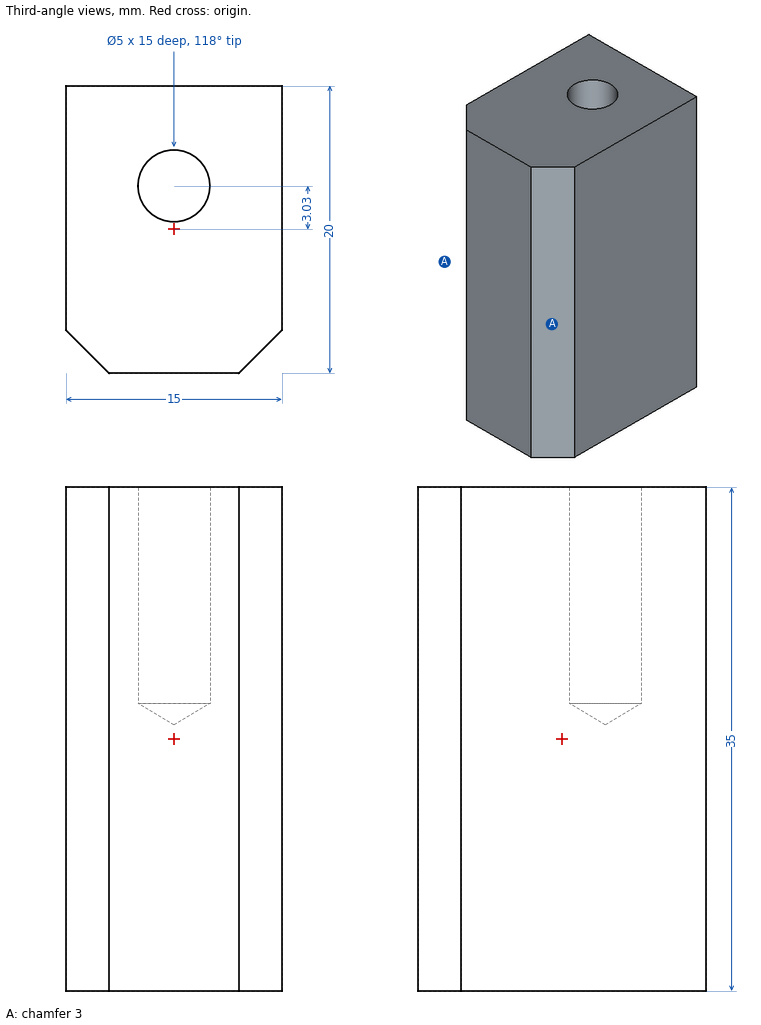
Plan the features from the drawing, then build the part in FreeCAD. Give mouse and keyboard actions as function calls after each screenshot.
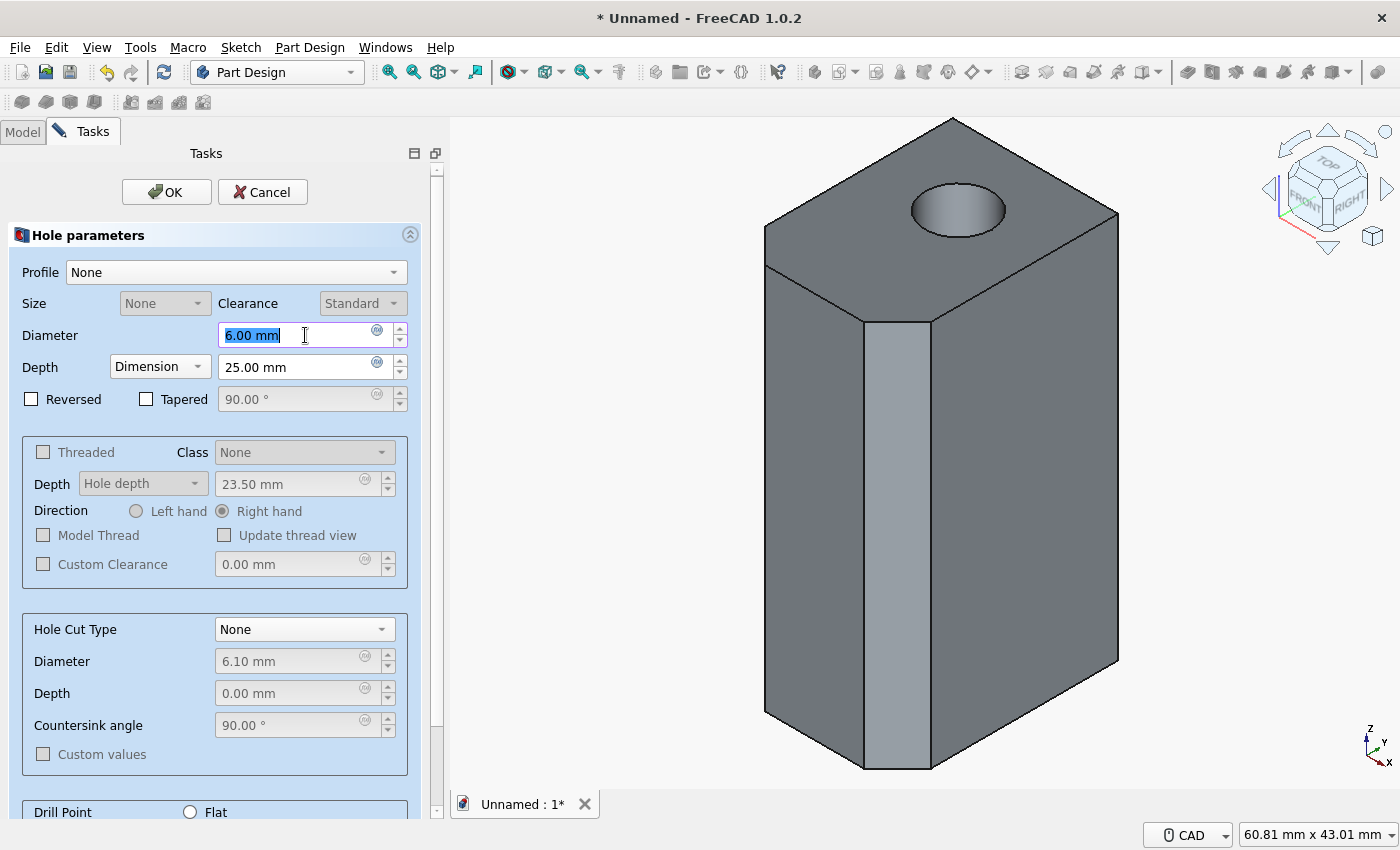
text(5)
key(Tab)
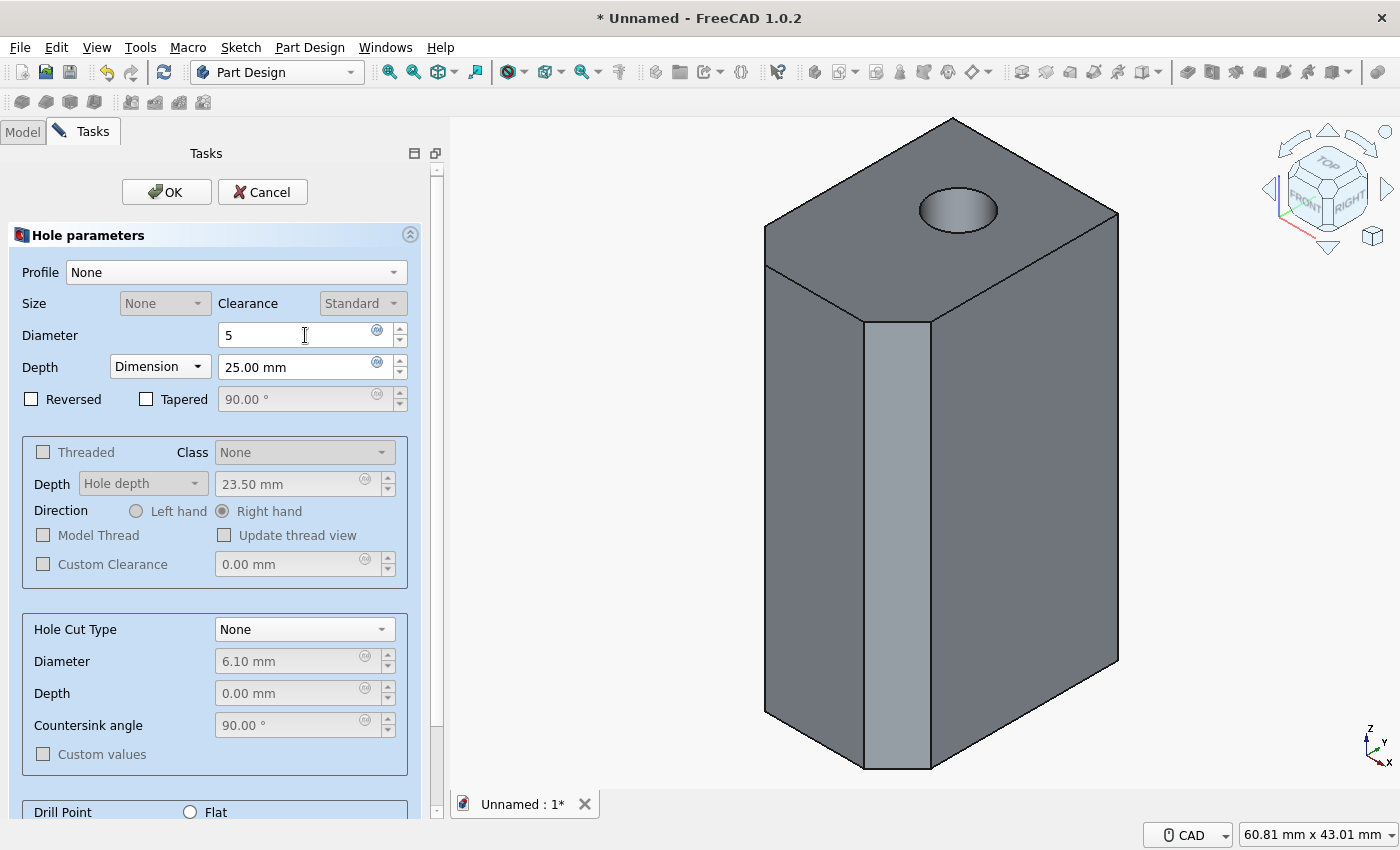
triple_click(305, 367)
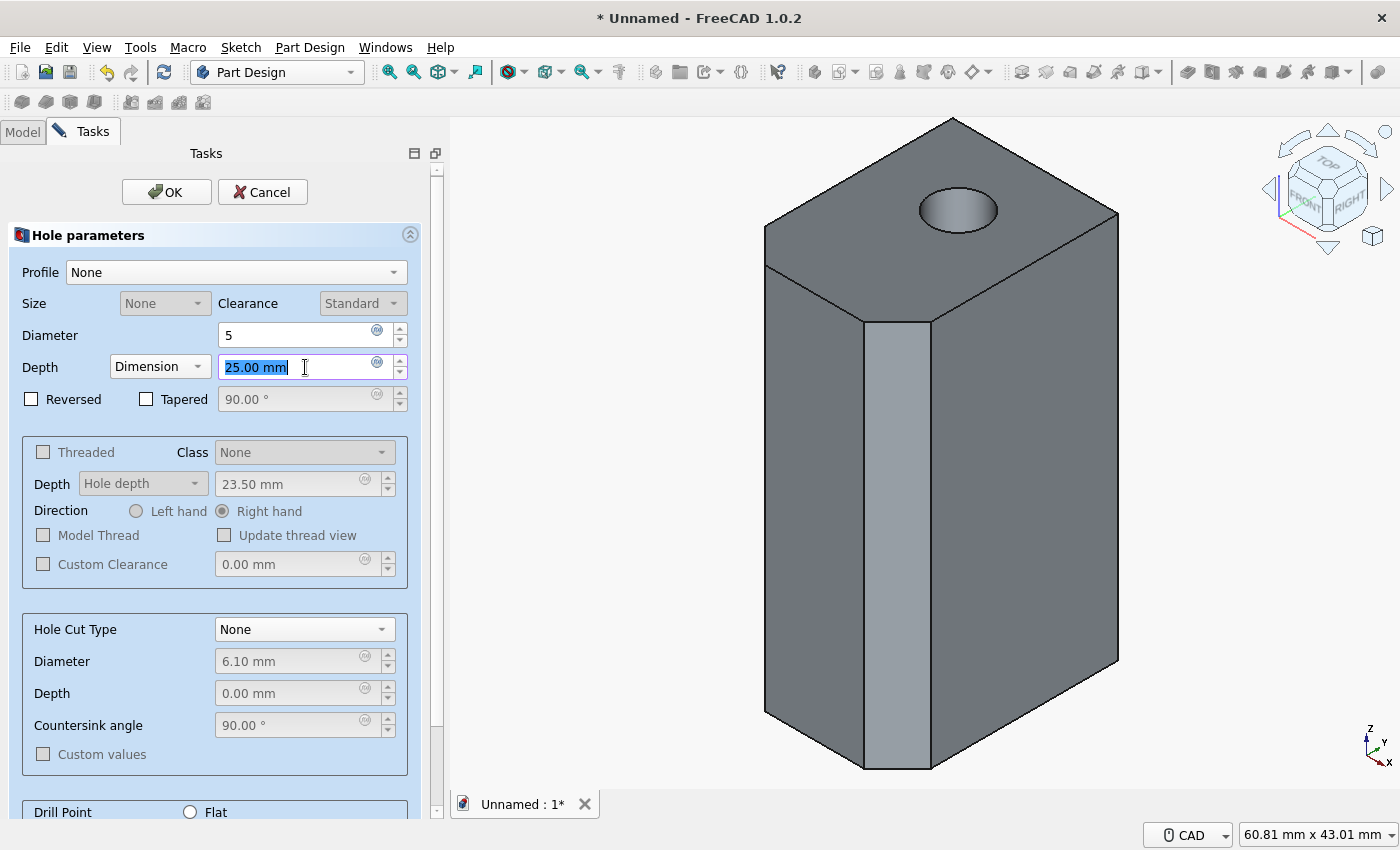
text(15)
key(Tab)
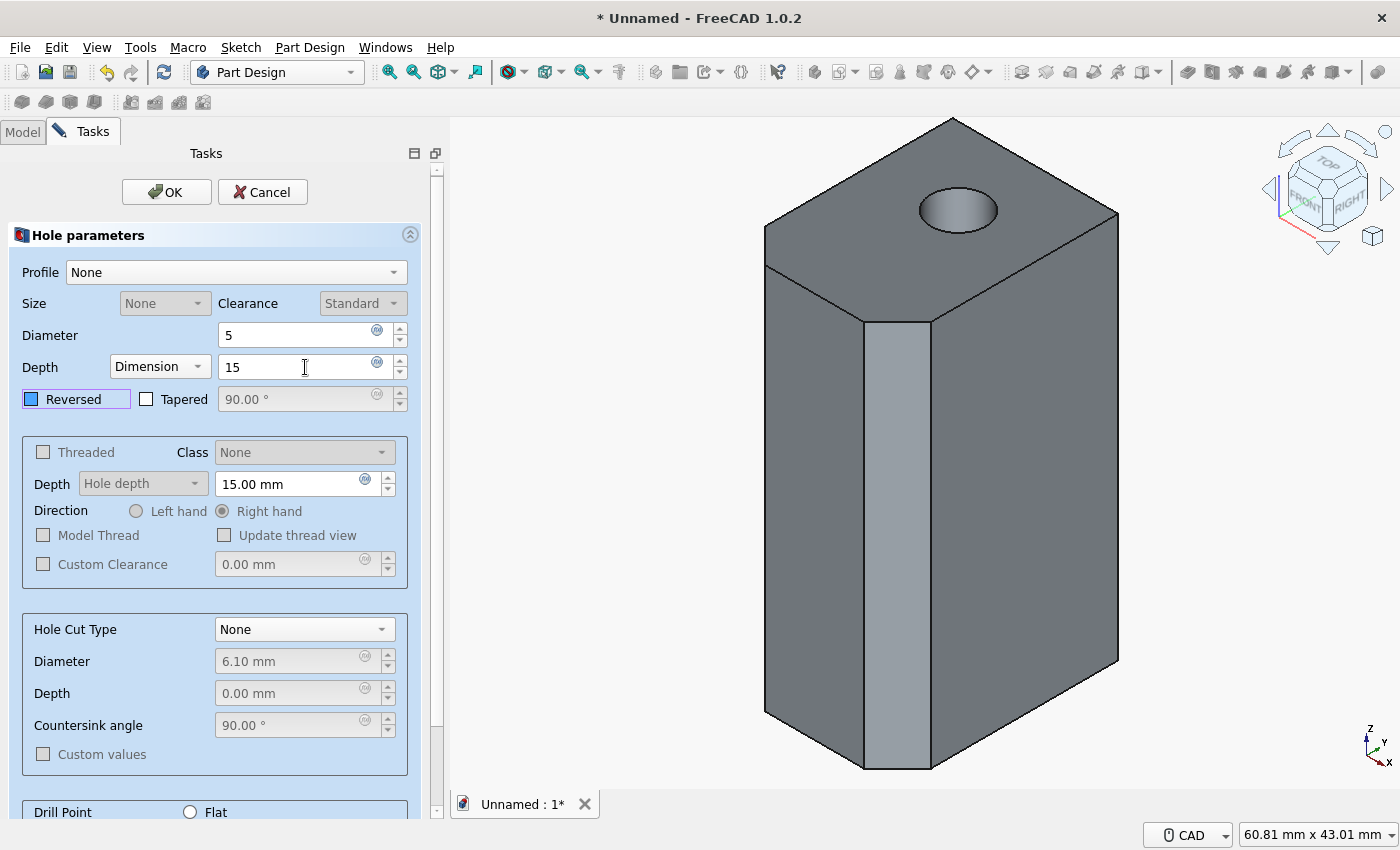
click(167, 192)